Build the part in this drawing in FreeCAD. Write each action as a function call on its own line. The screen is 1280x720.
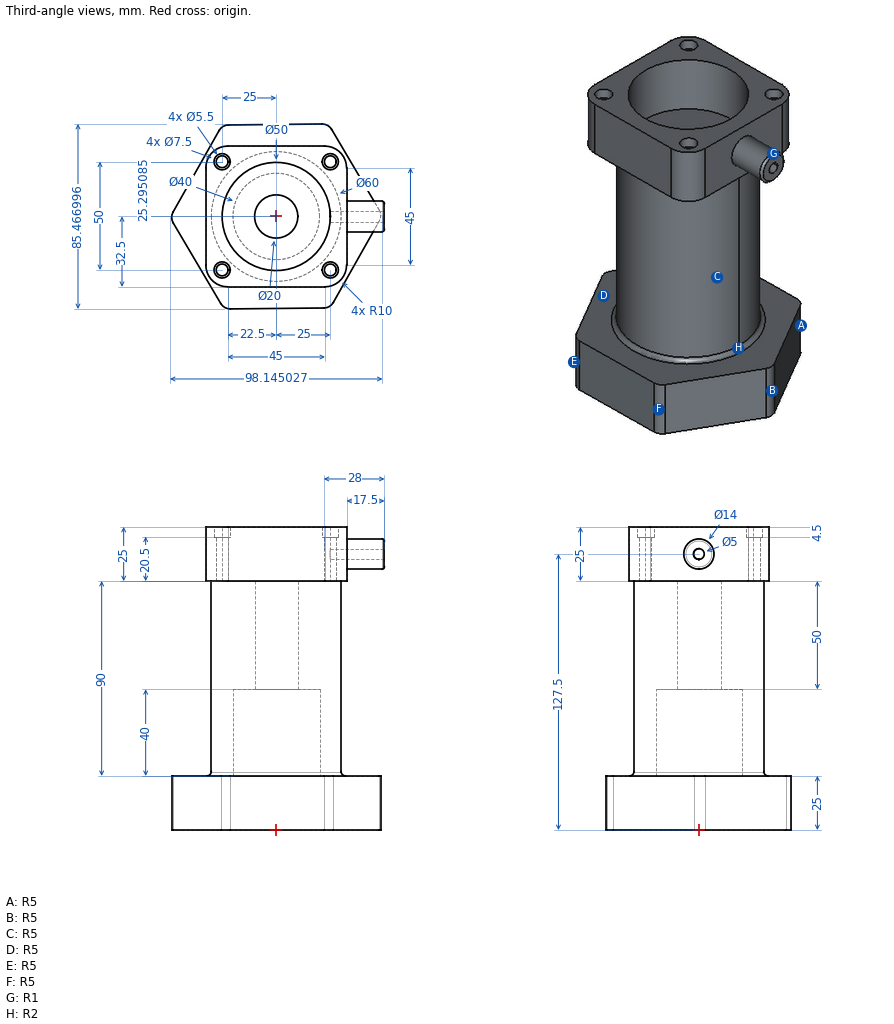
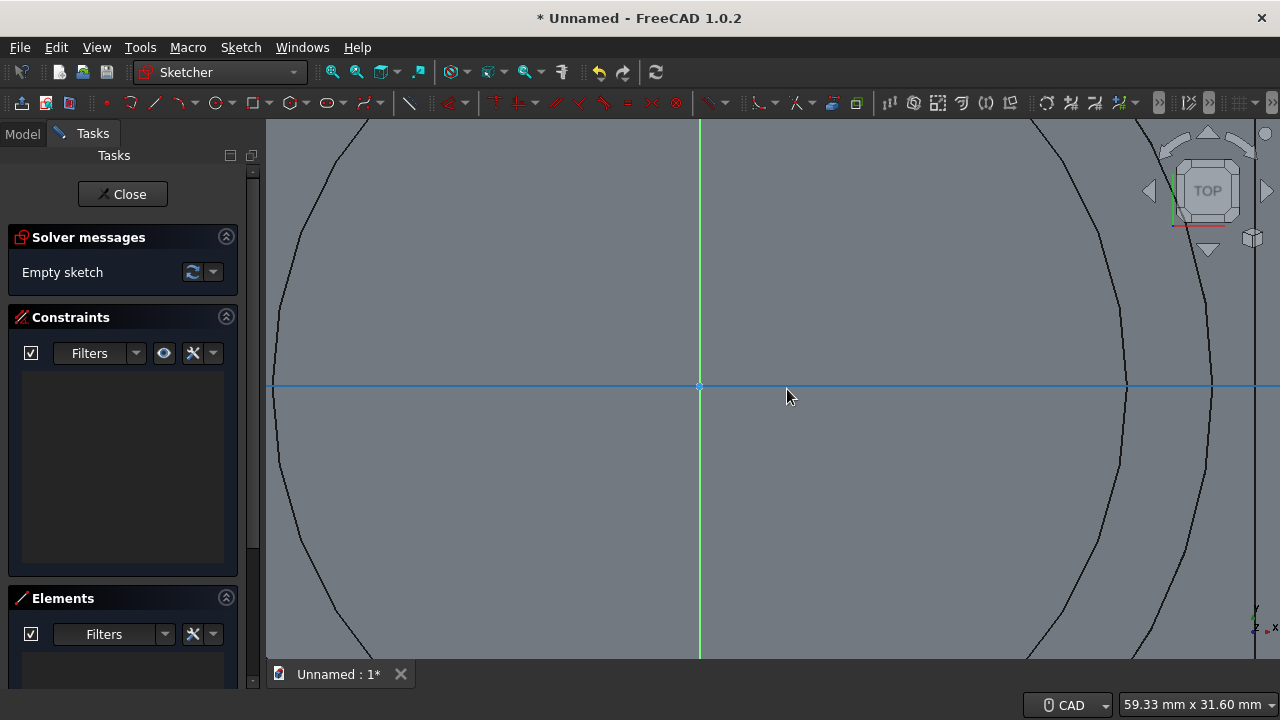
click(216, 104)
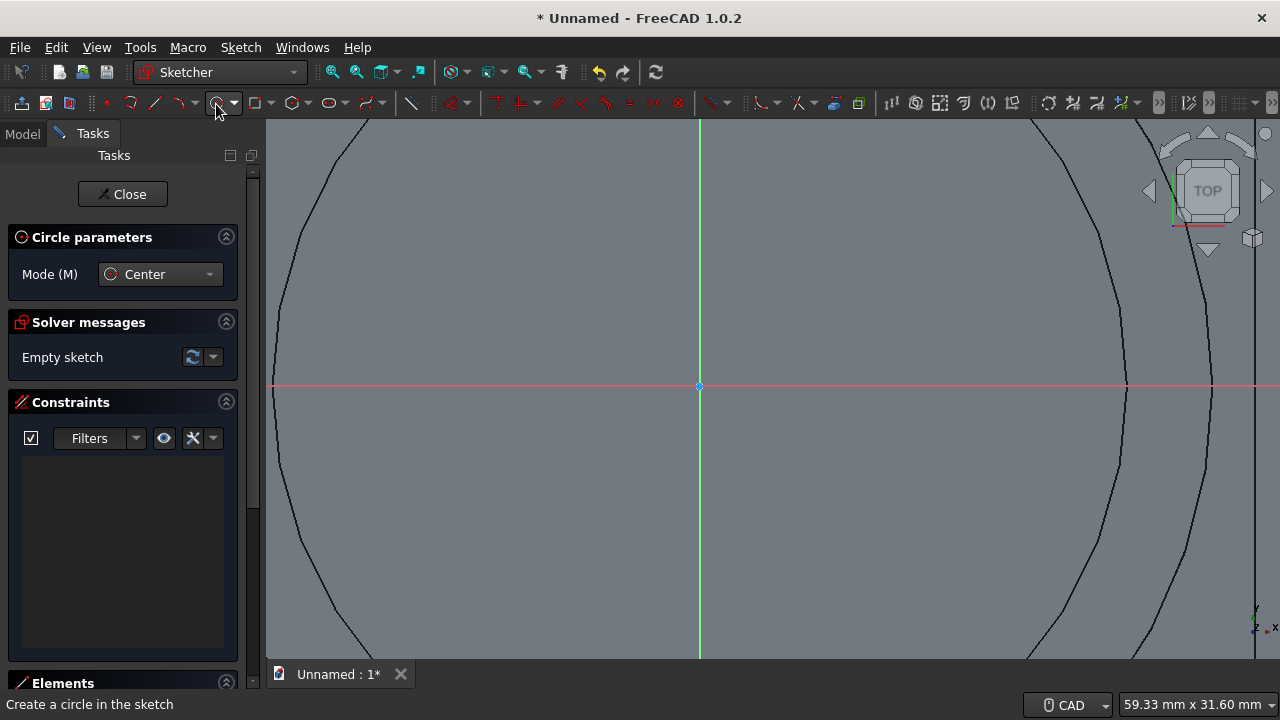
click(700, 386)
click(821, 266)
key(Escape)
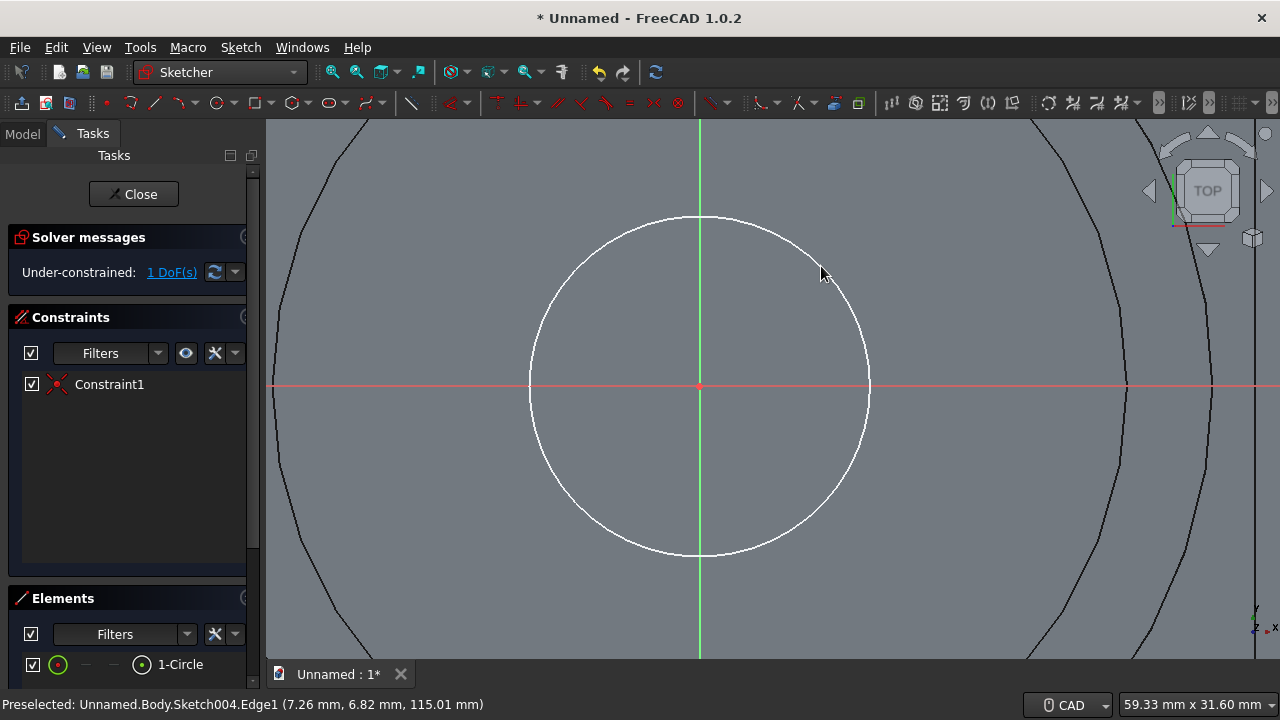
click(450, 104)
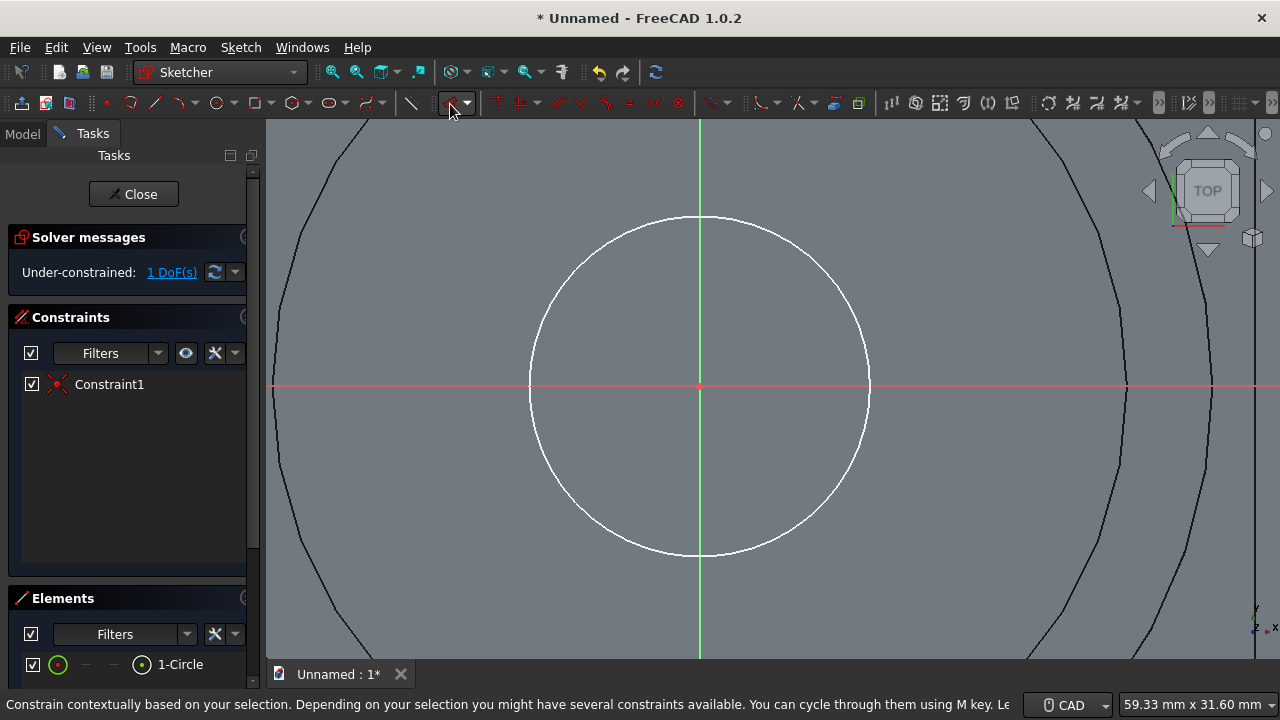
click(820, 266)
click(843, 243)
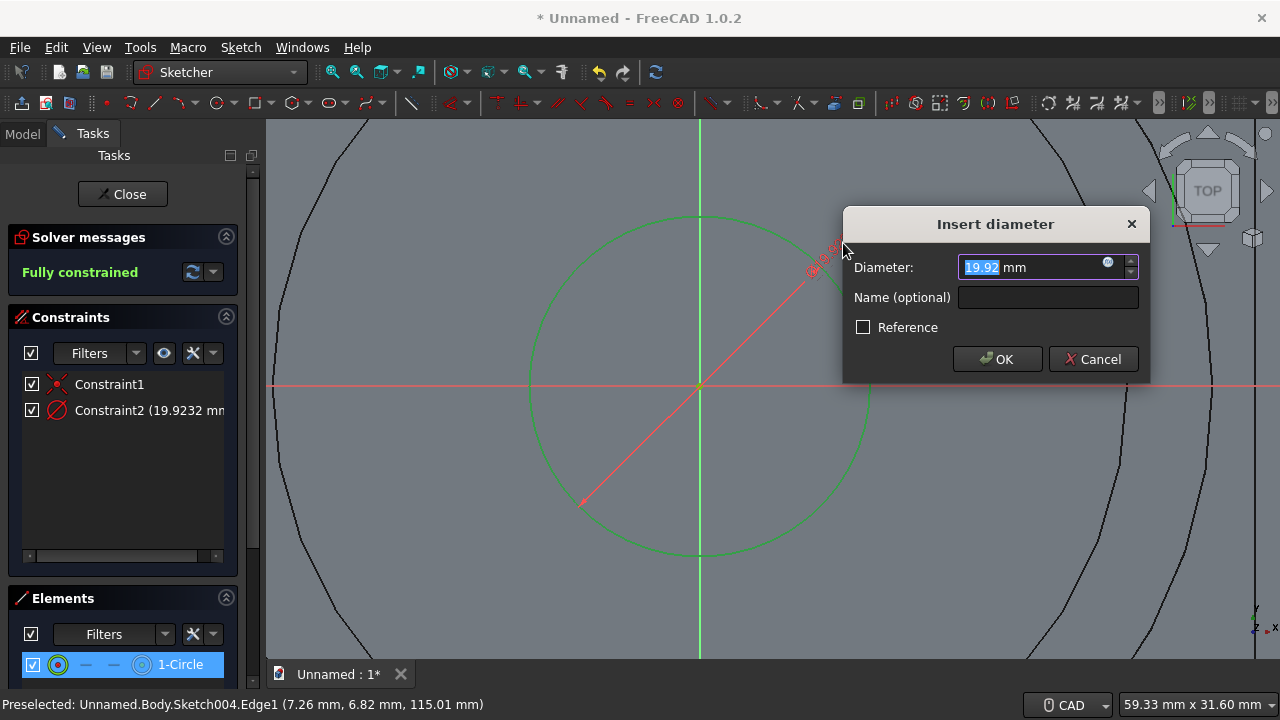
text(20)
key(Return)
key(Escape)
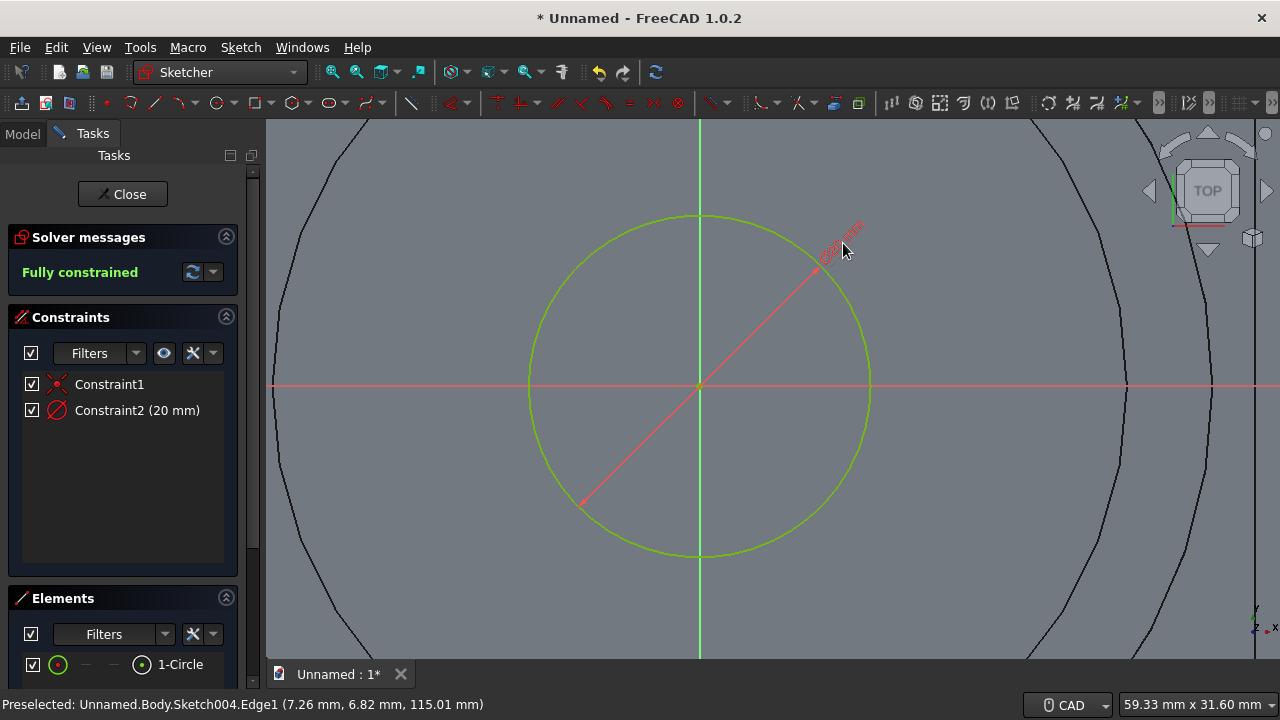
click(123, 194)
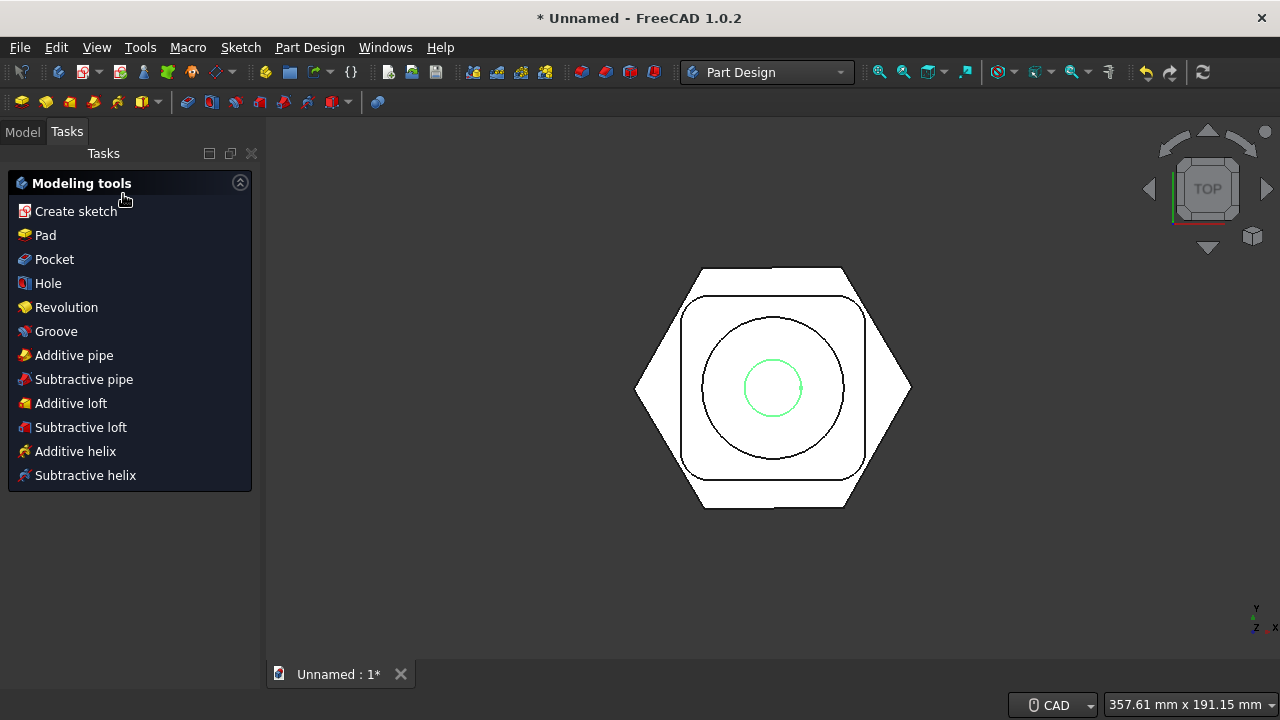
click(188, 102)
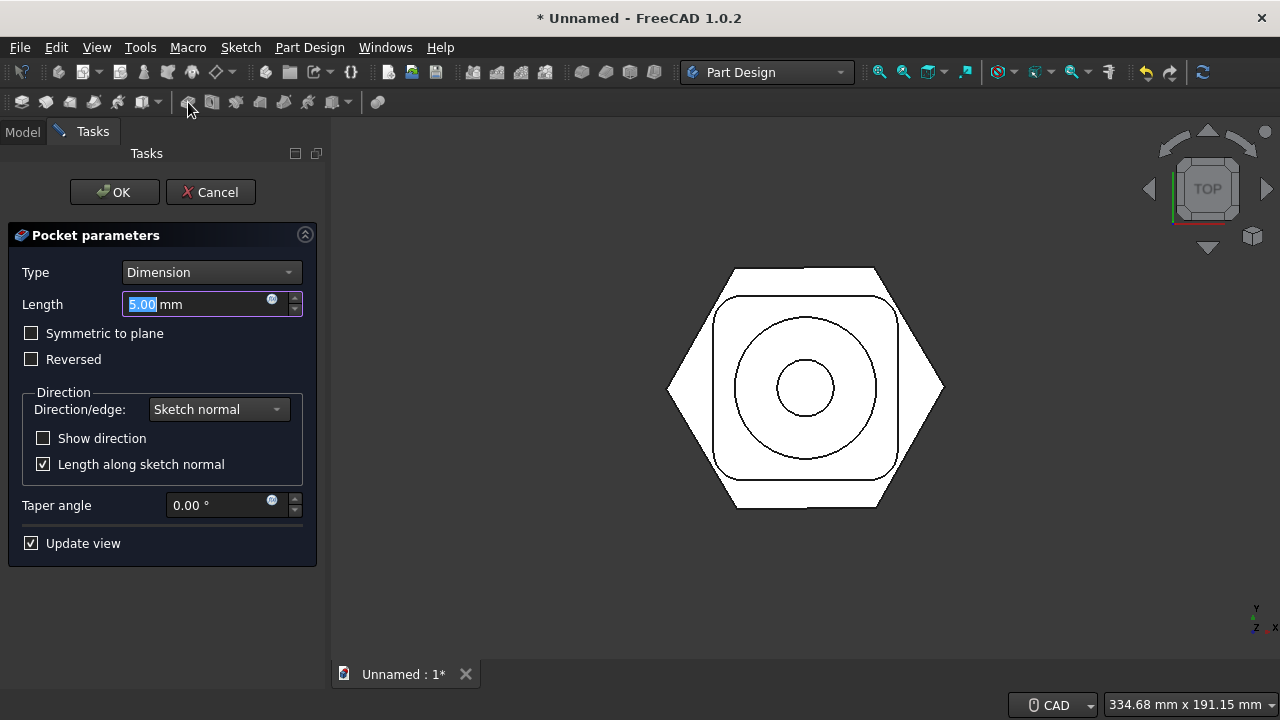
text(50)
key(Tab)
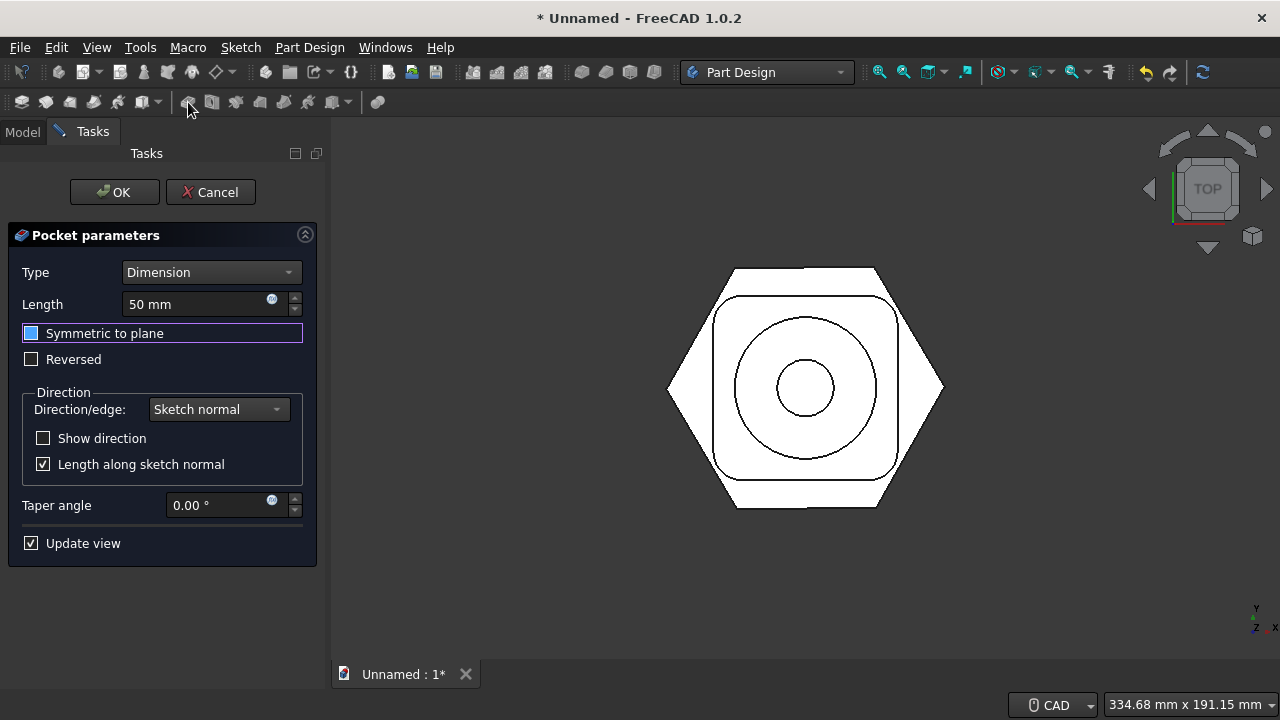
click(115, 192)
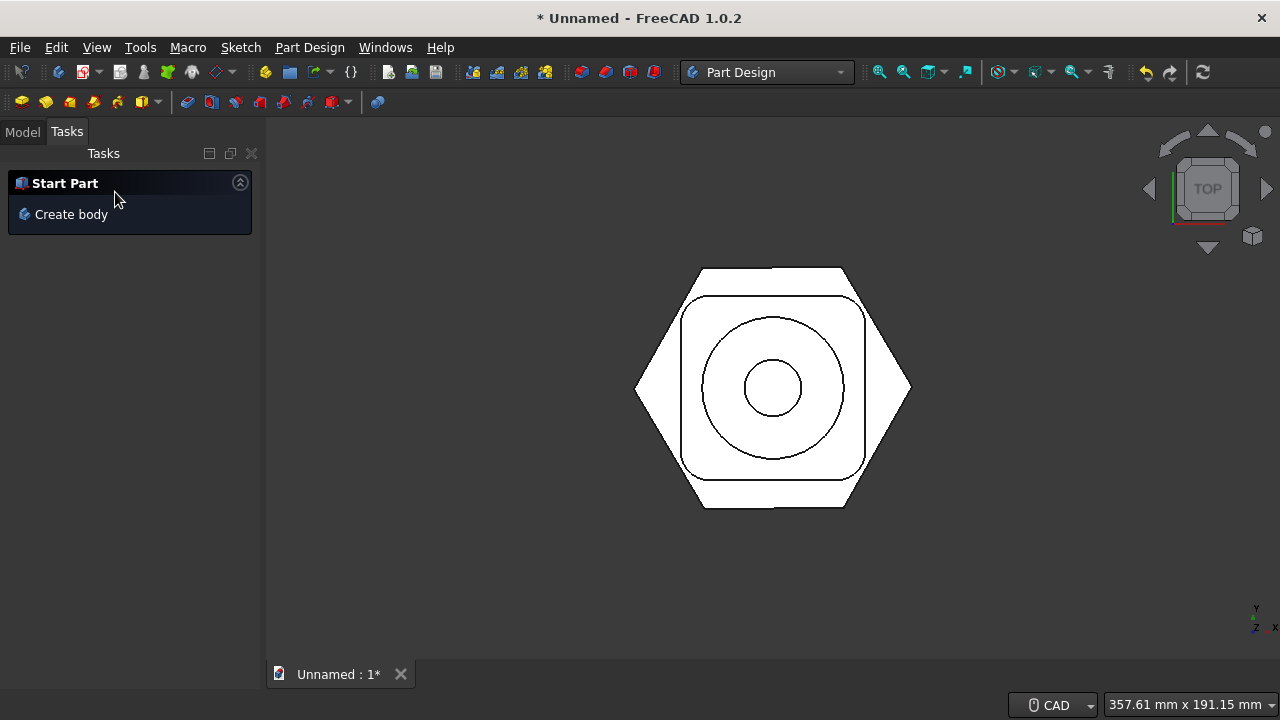
click(880, 72)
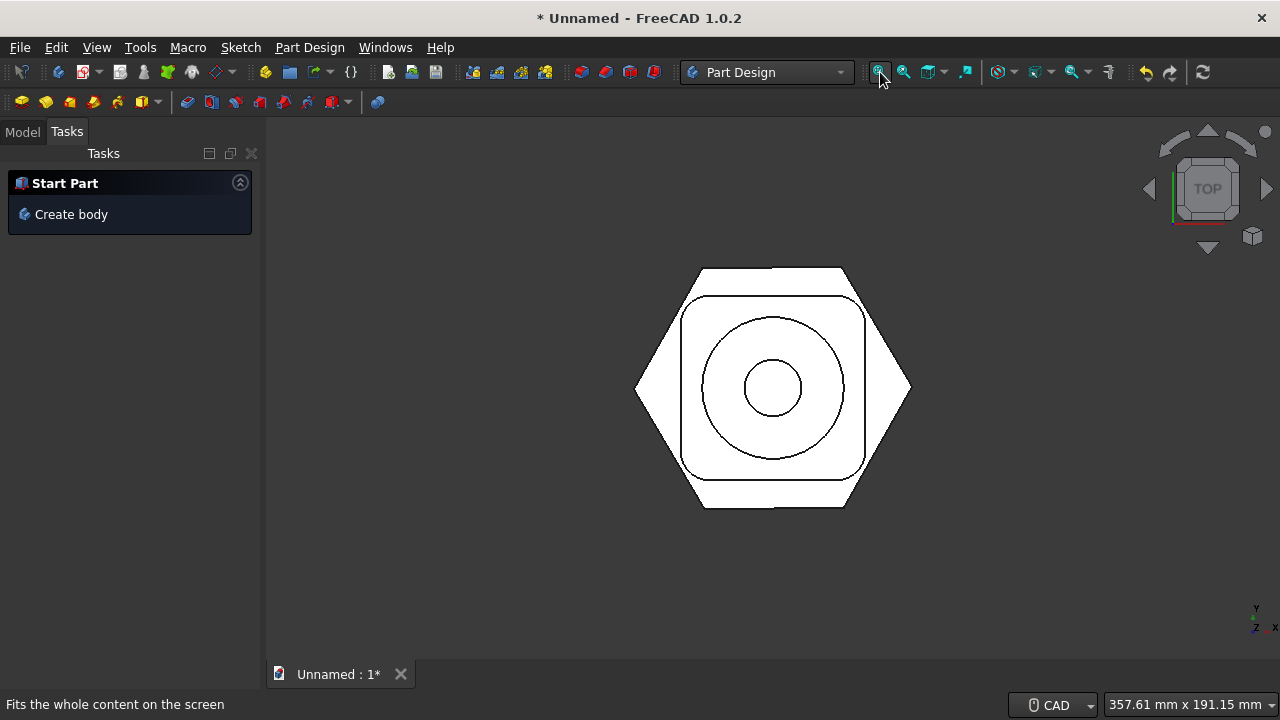
click(773, 387)